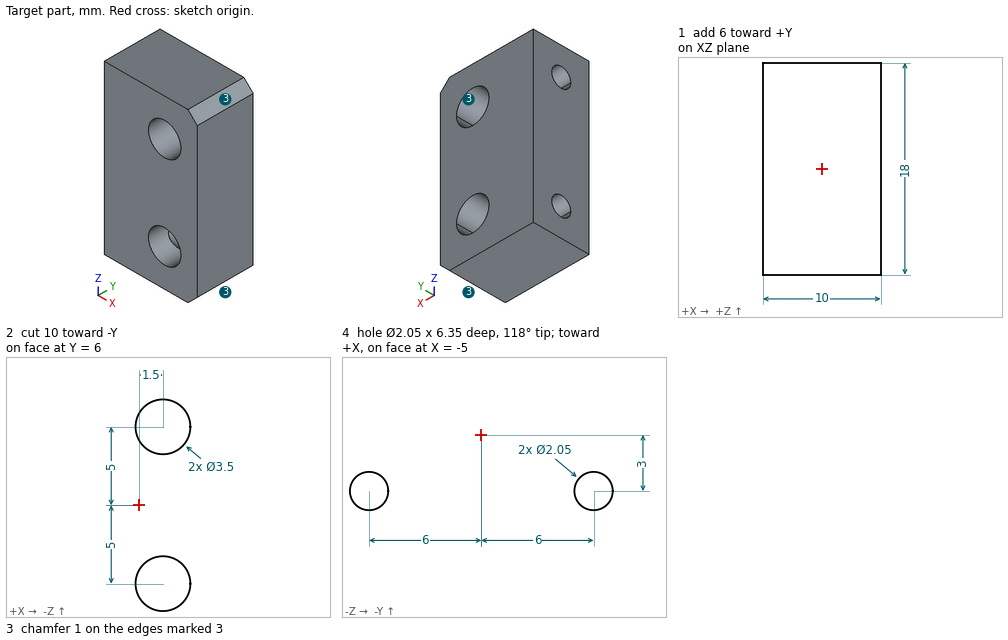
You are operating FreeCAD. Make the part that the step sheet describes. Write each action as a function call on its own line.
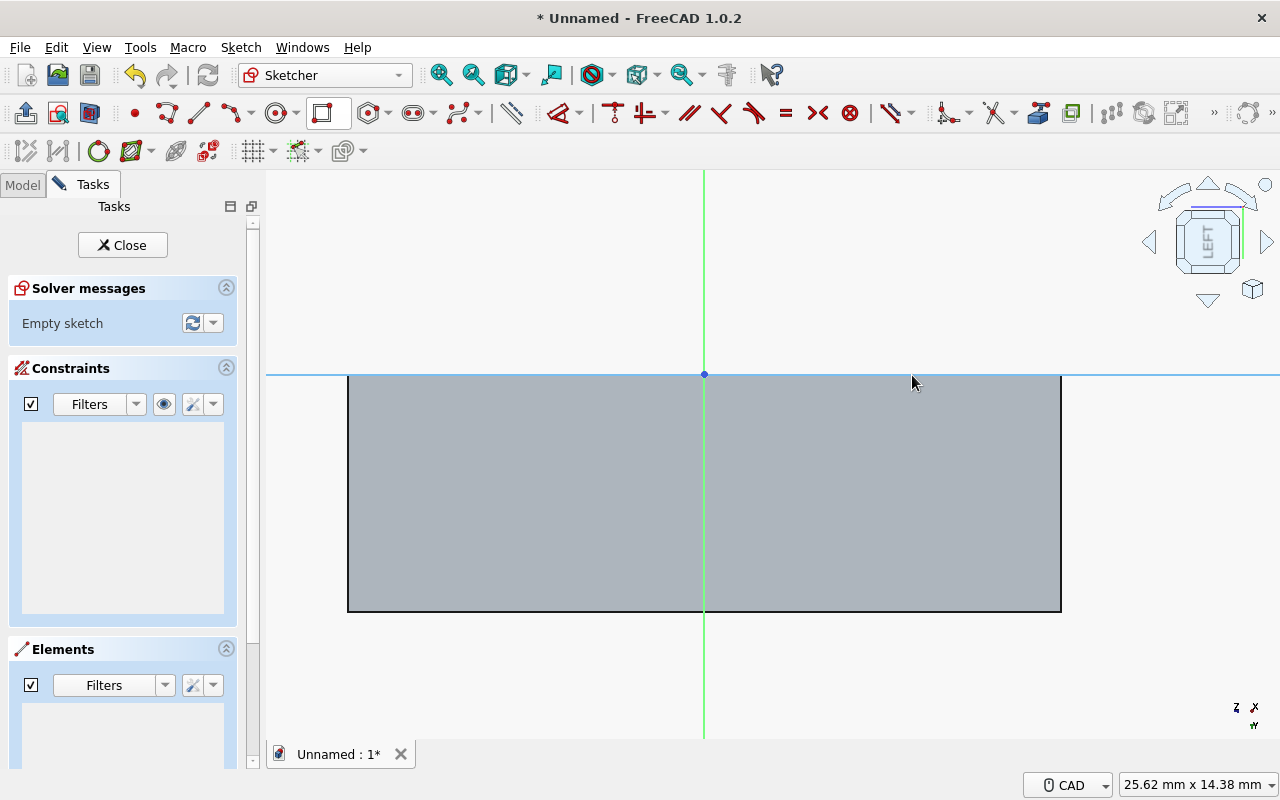
key(g)
key(c)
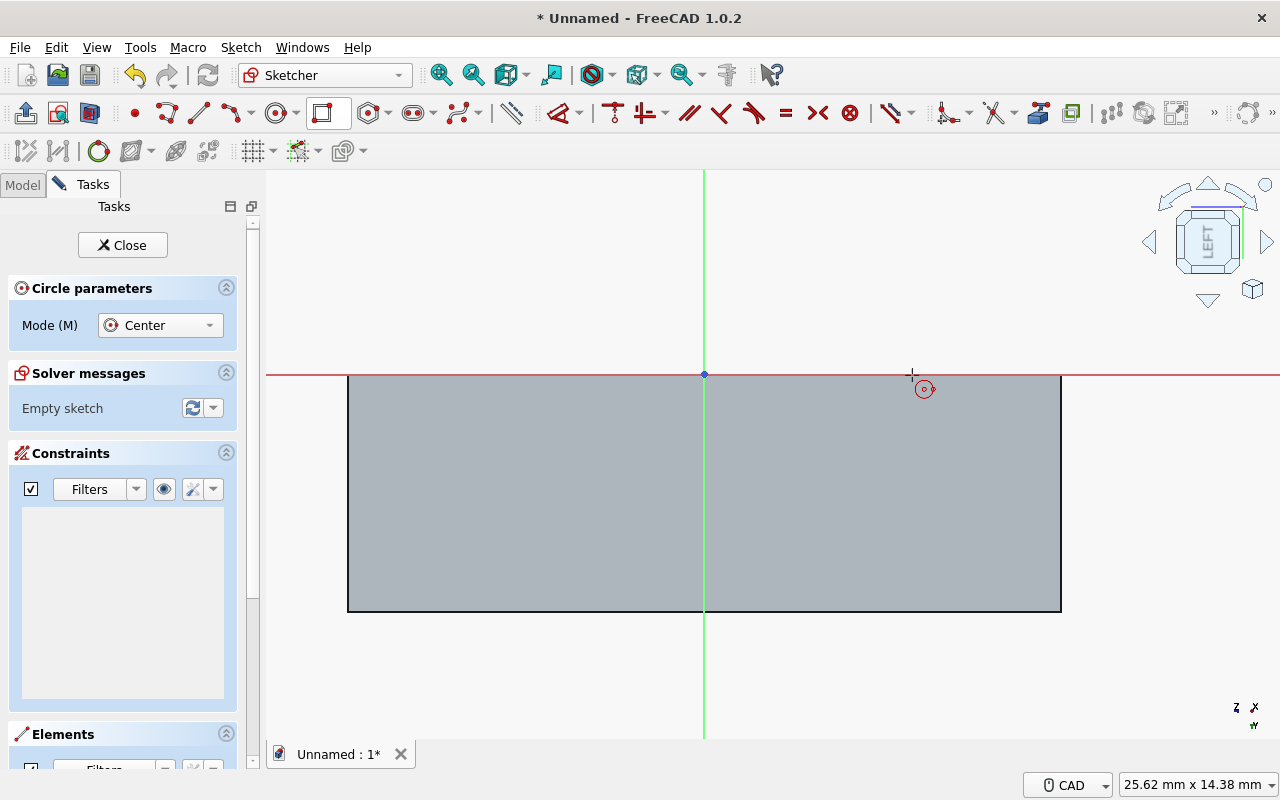
click(942, 493)
move(970, 465)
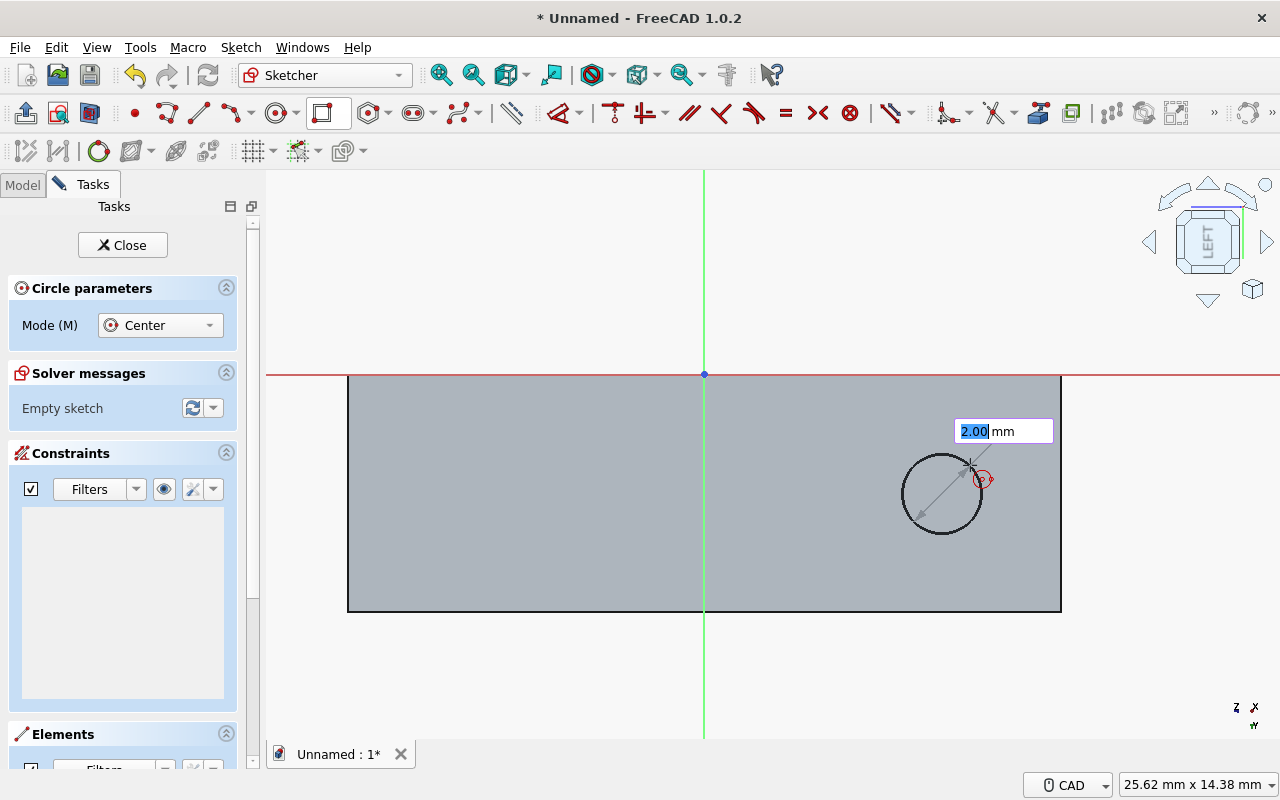
text(2.05)
key(Return)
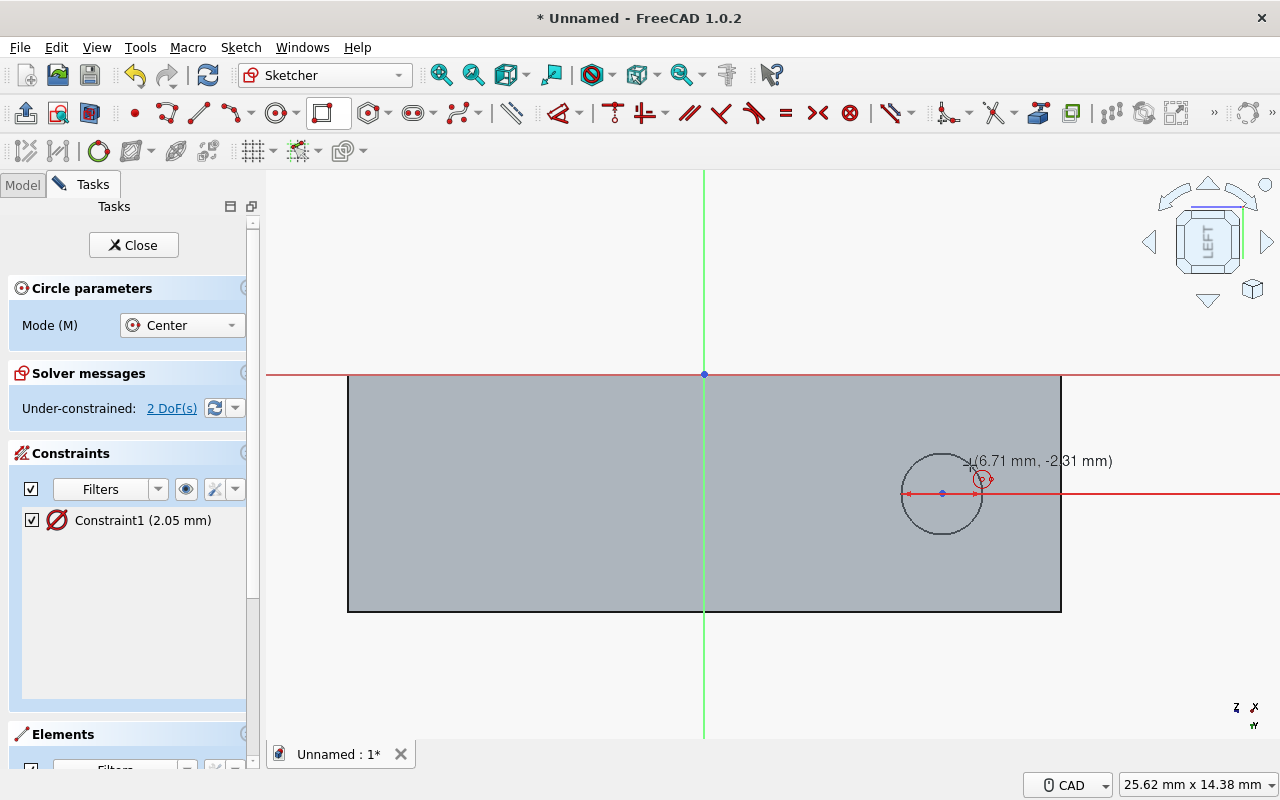
click(467, 493)
move(496, 465)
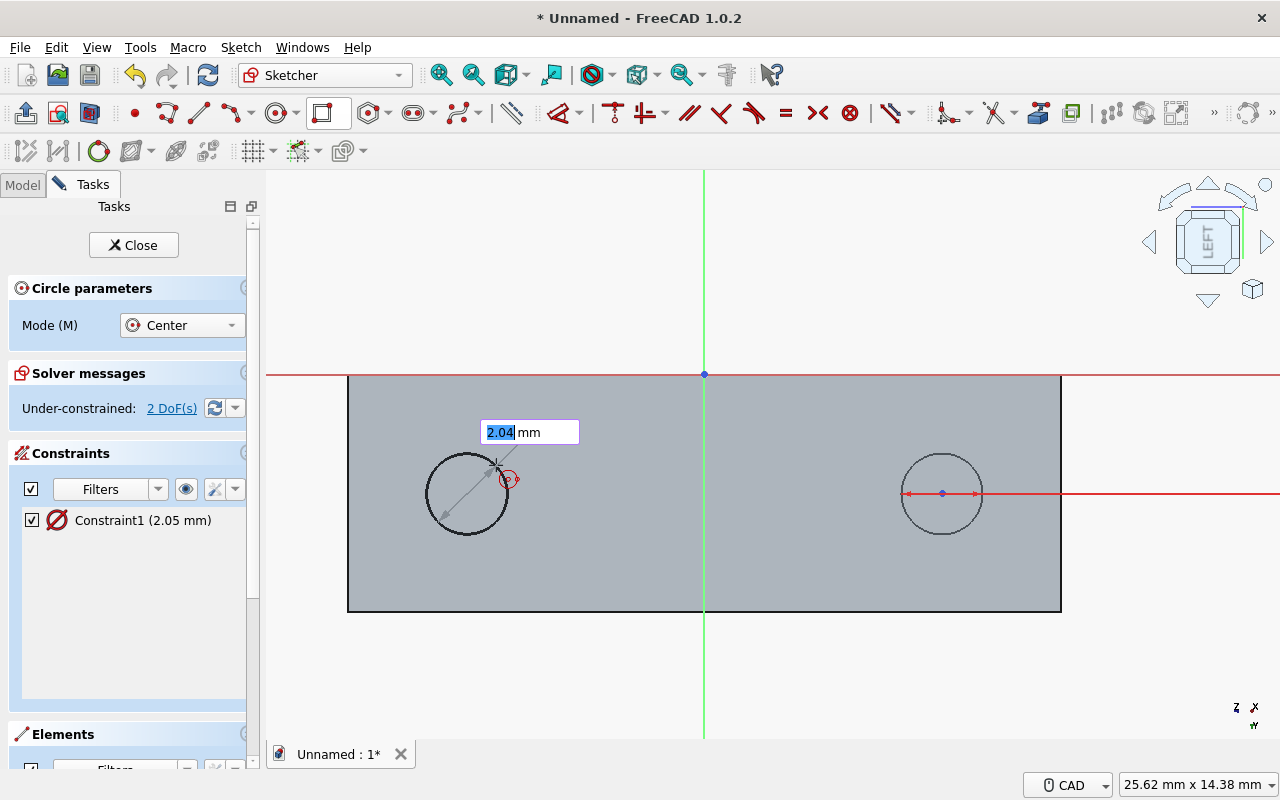
text(2.05)
key(Return)
key(Escape)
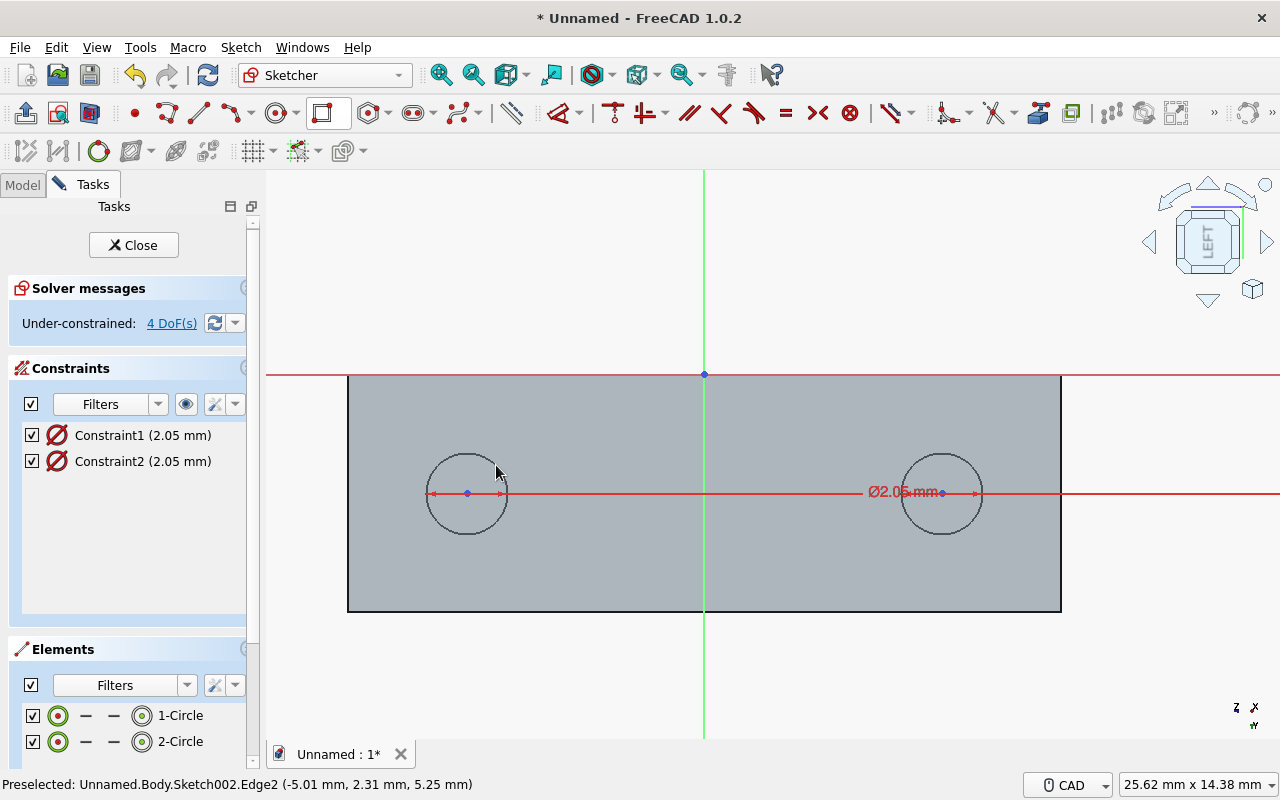
click(942, 494)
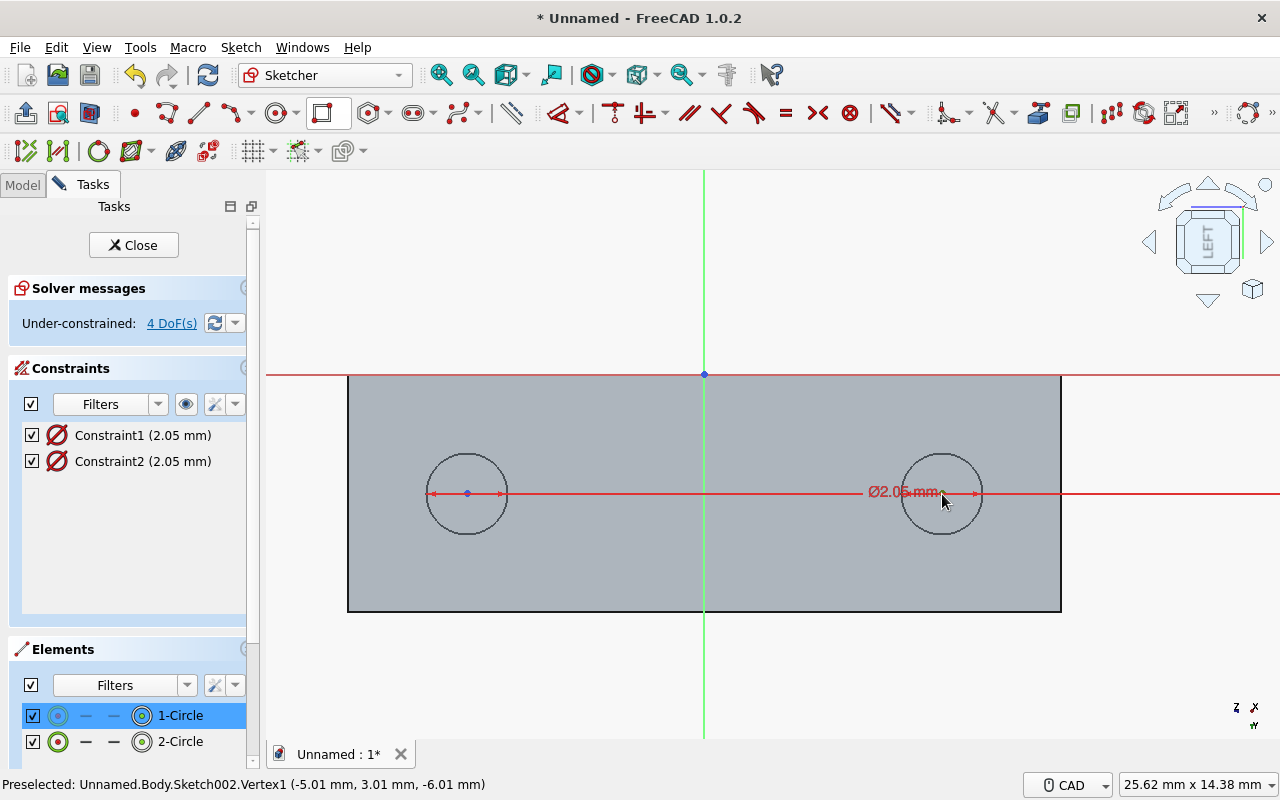
click(467, 494)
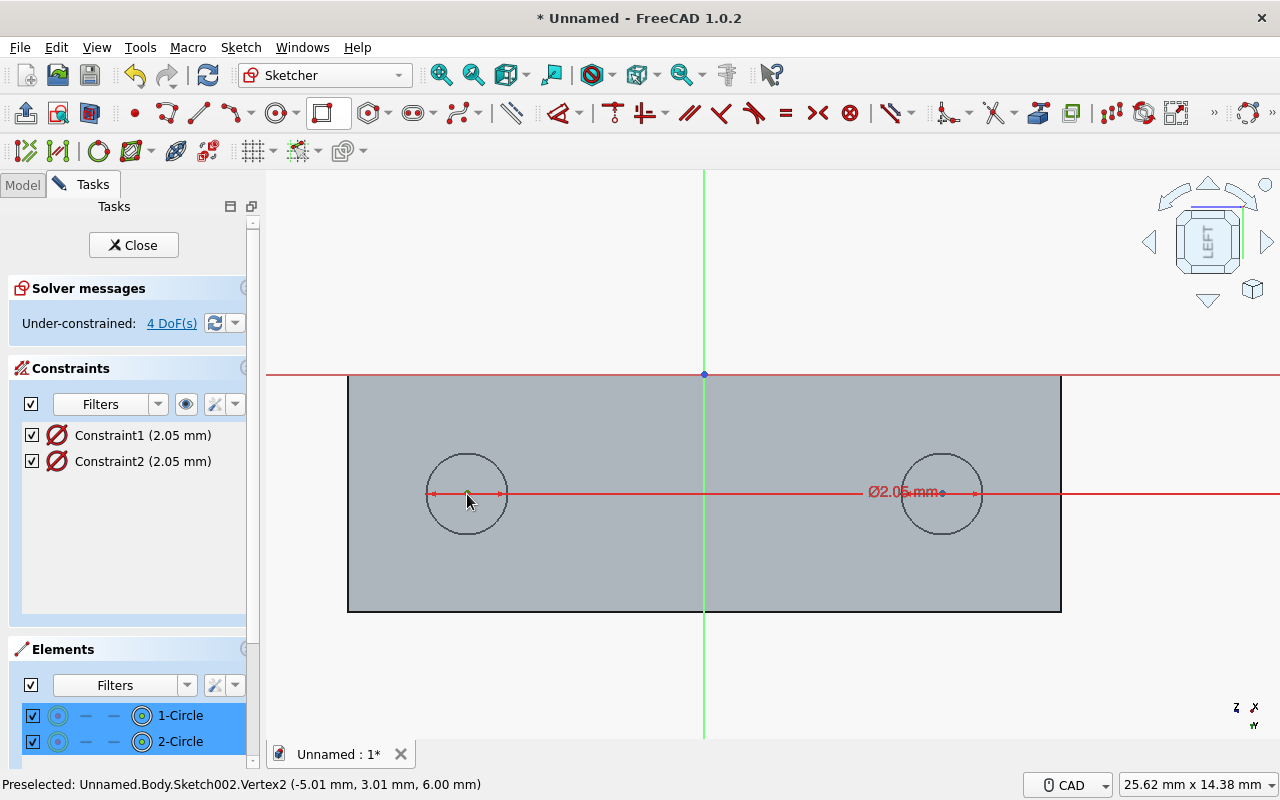
key(h)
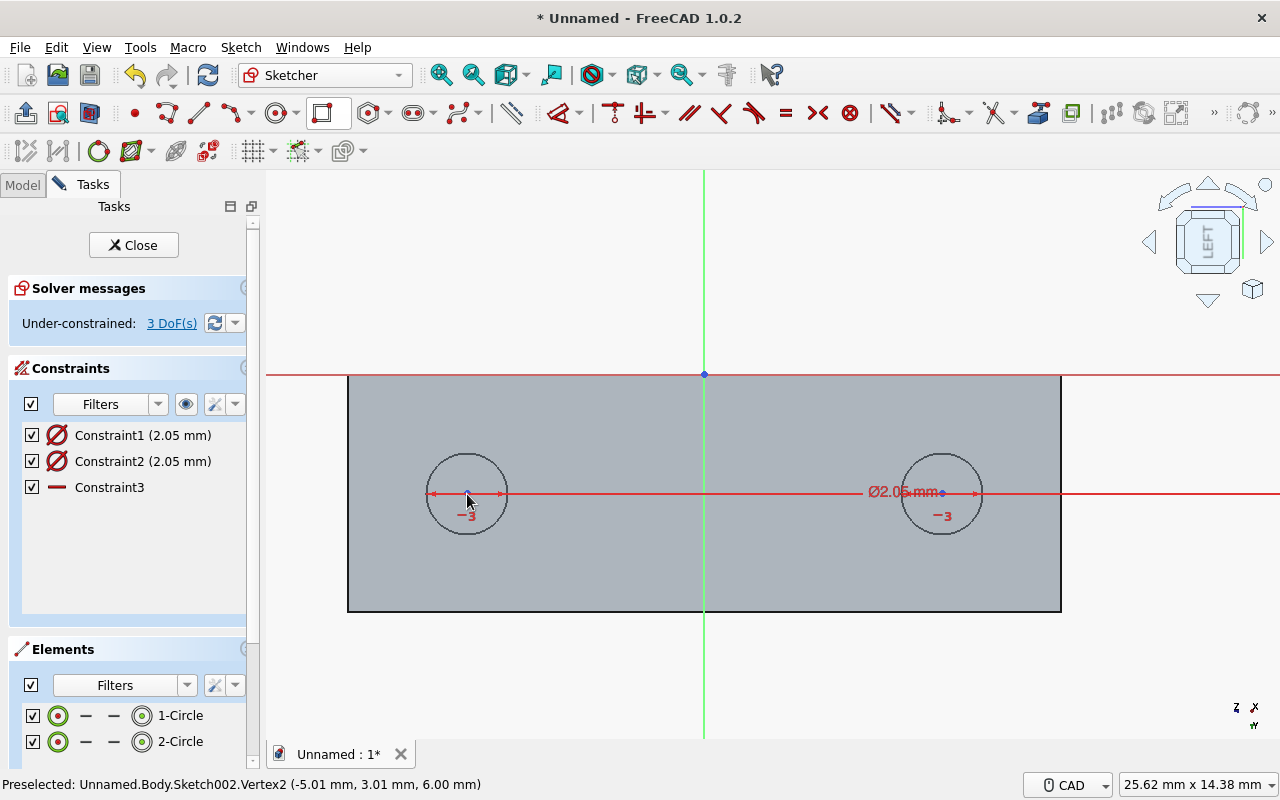
click(558, 114)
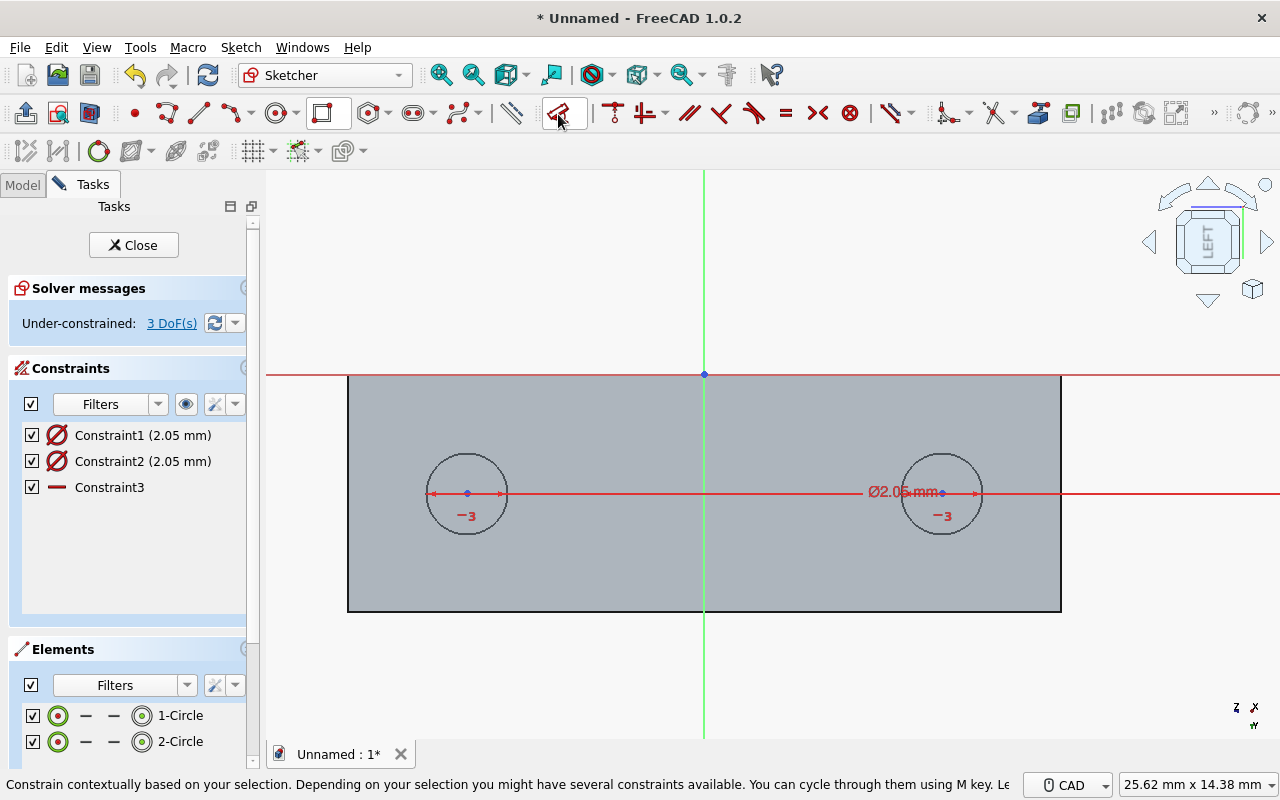
click(942, 494)
click(823, 341)